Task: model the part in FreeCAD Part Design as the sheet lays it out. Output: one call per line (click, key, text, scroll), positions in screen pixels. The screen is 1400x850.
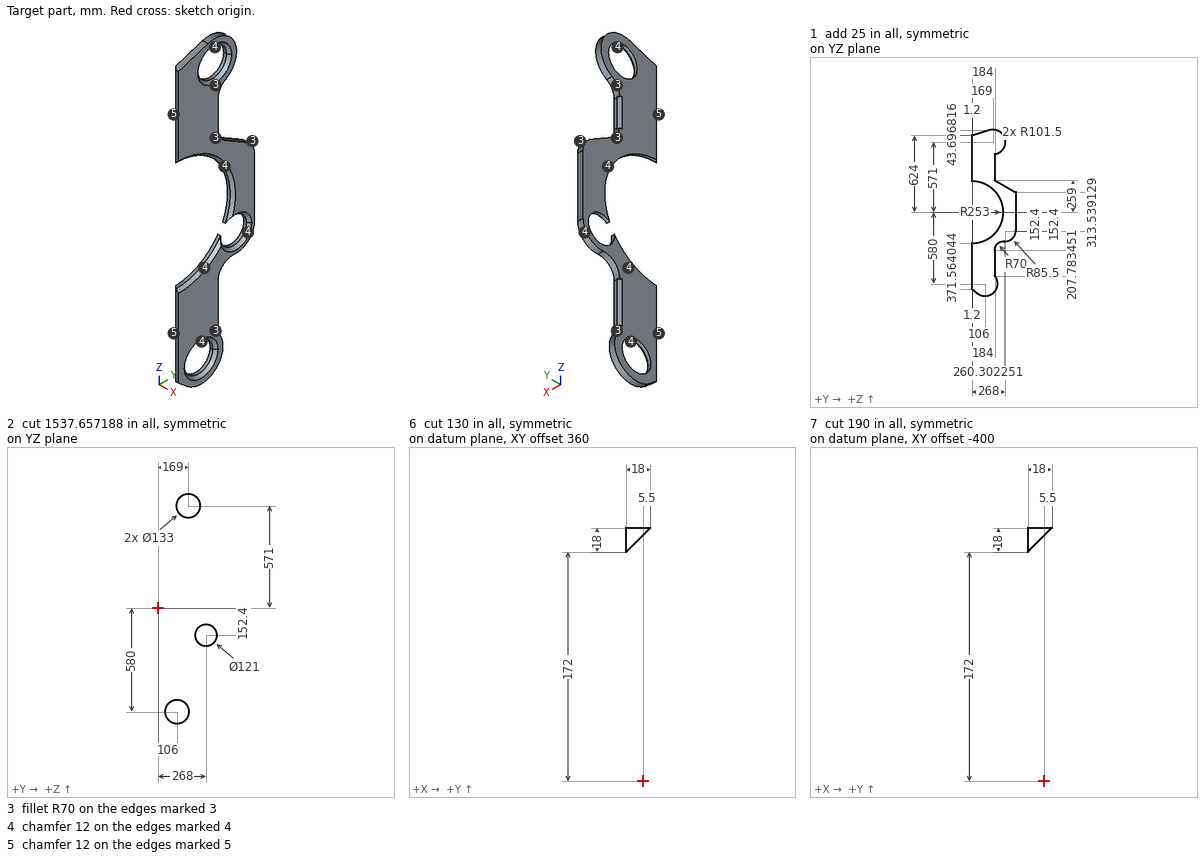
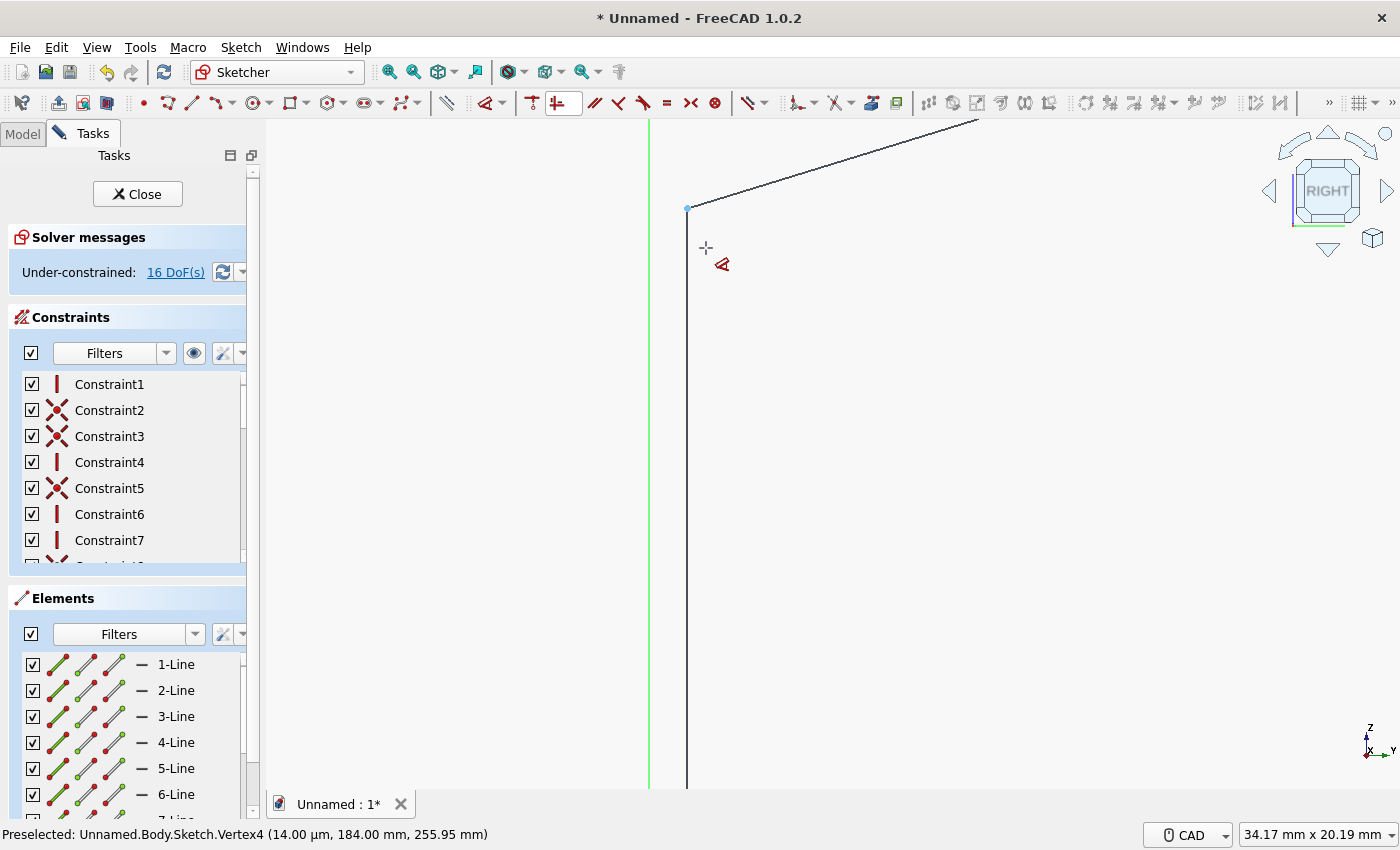
click(687, 209)
click(668, 175)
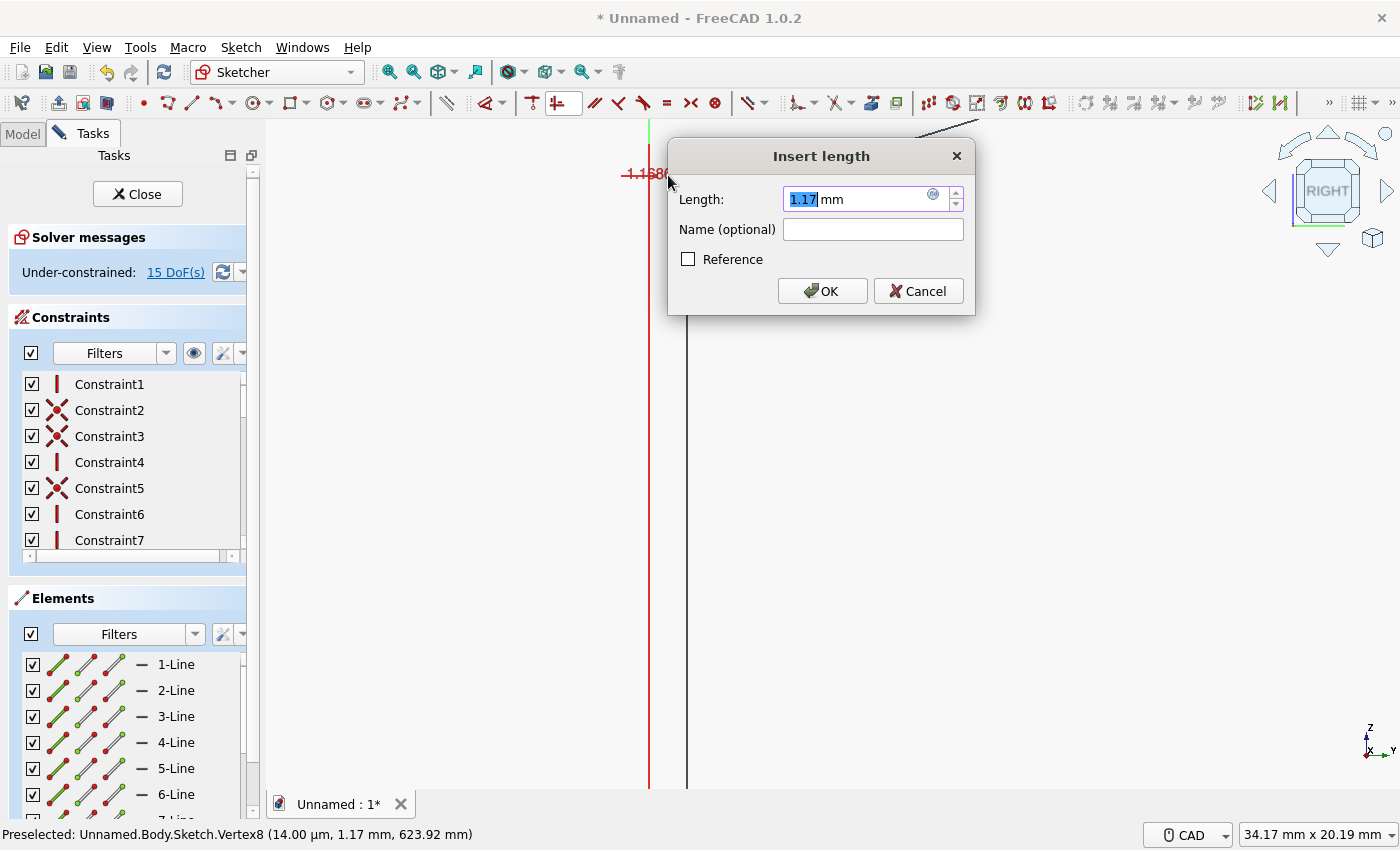
text(1.2)
key(Return)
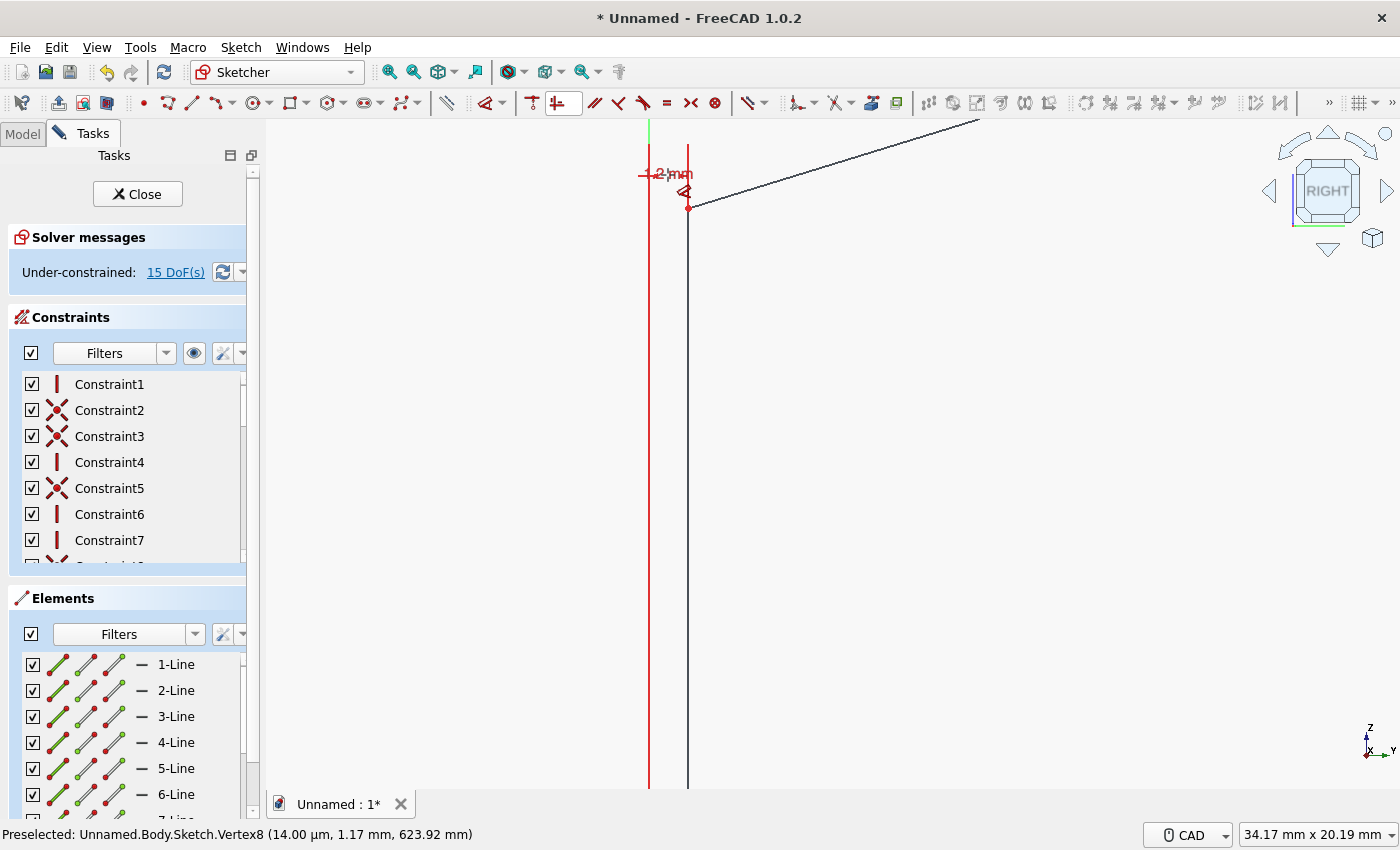
scroll(764, 454, down, 15)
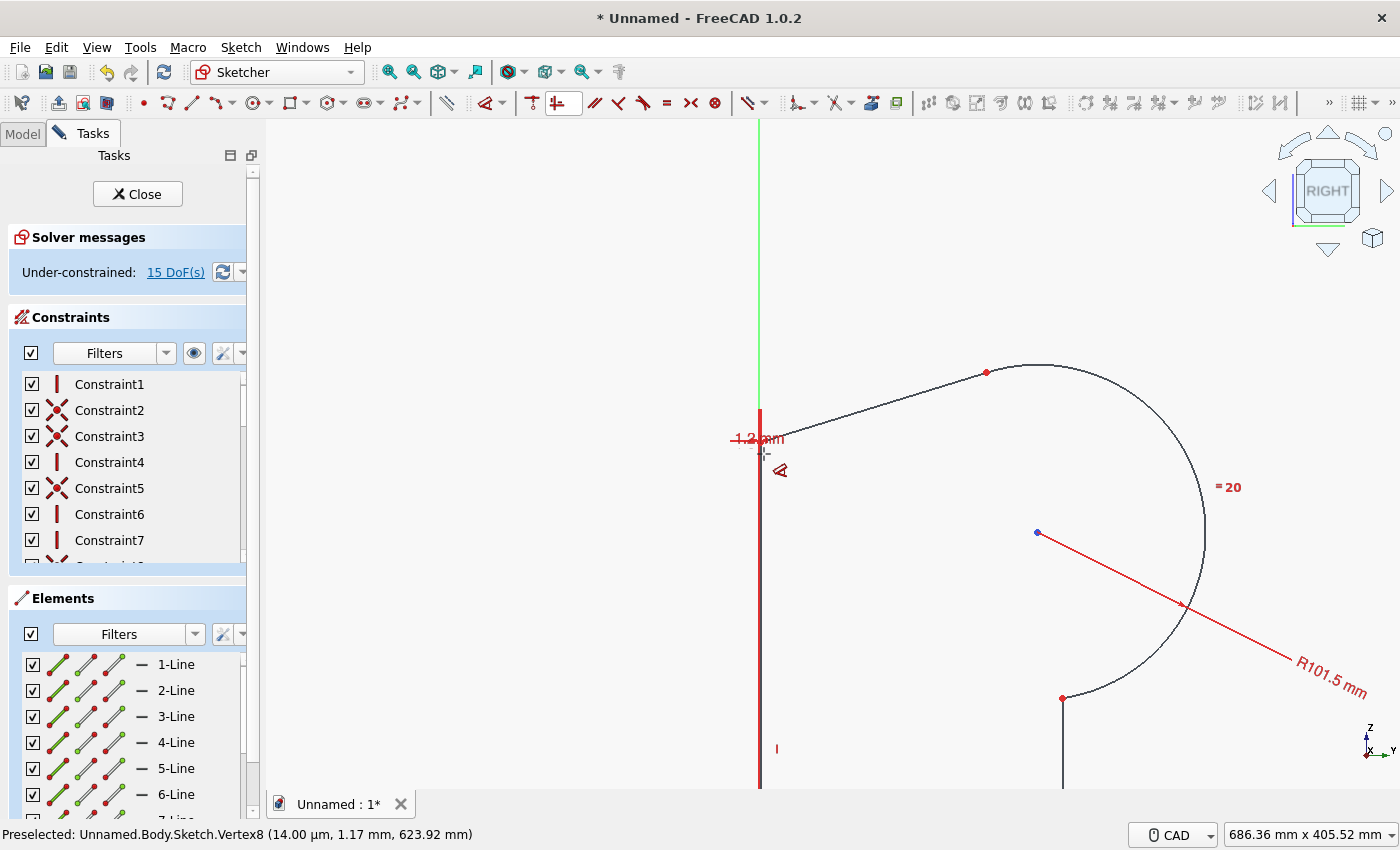
scroll(692, 198, down, 8)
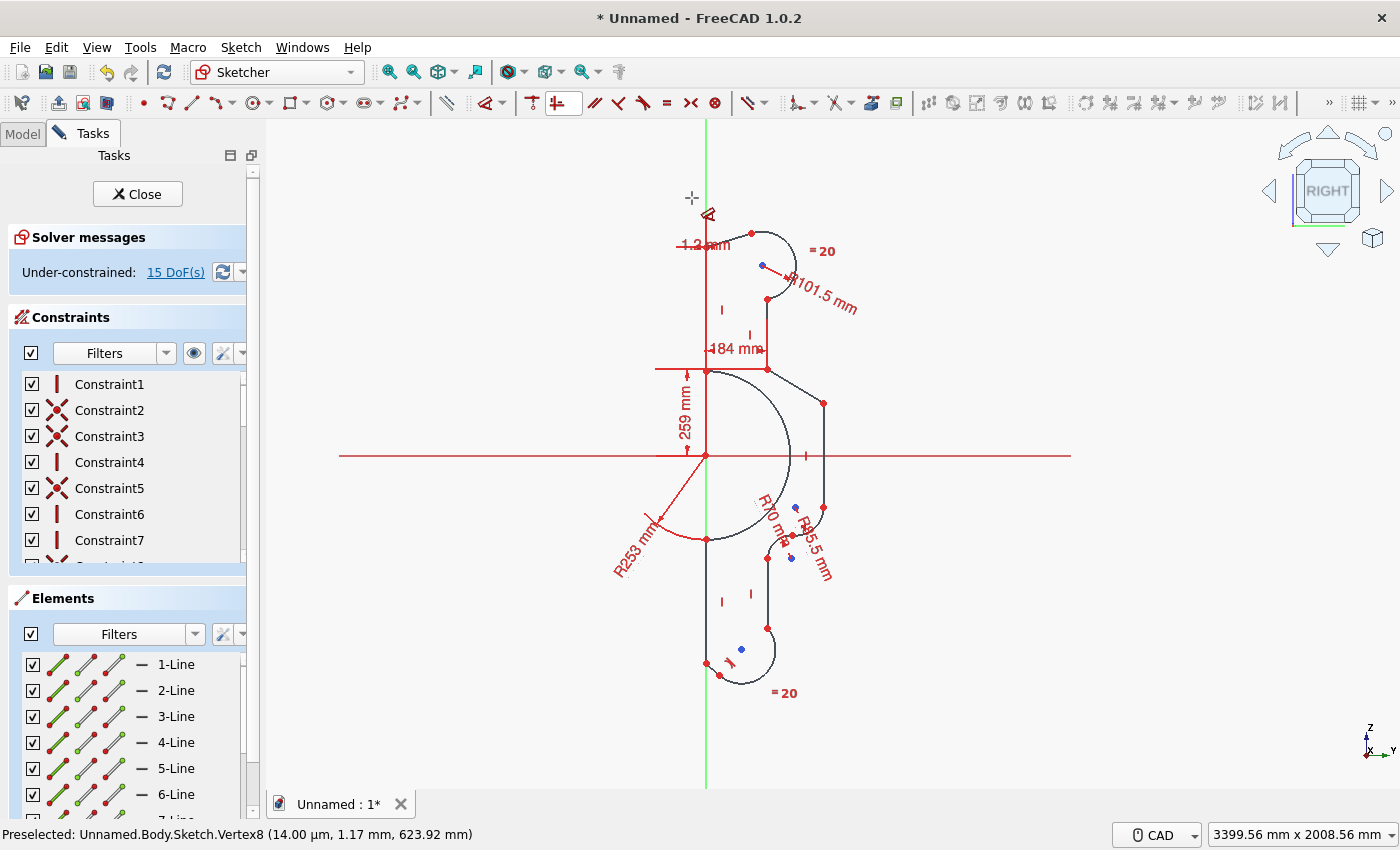
click(706, 247)
click(672, 304)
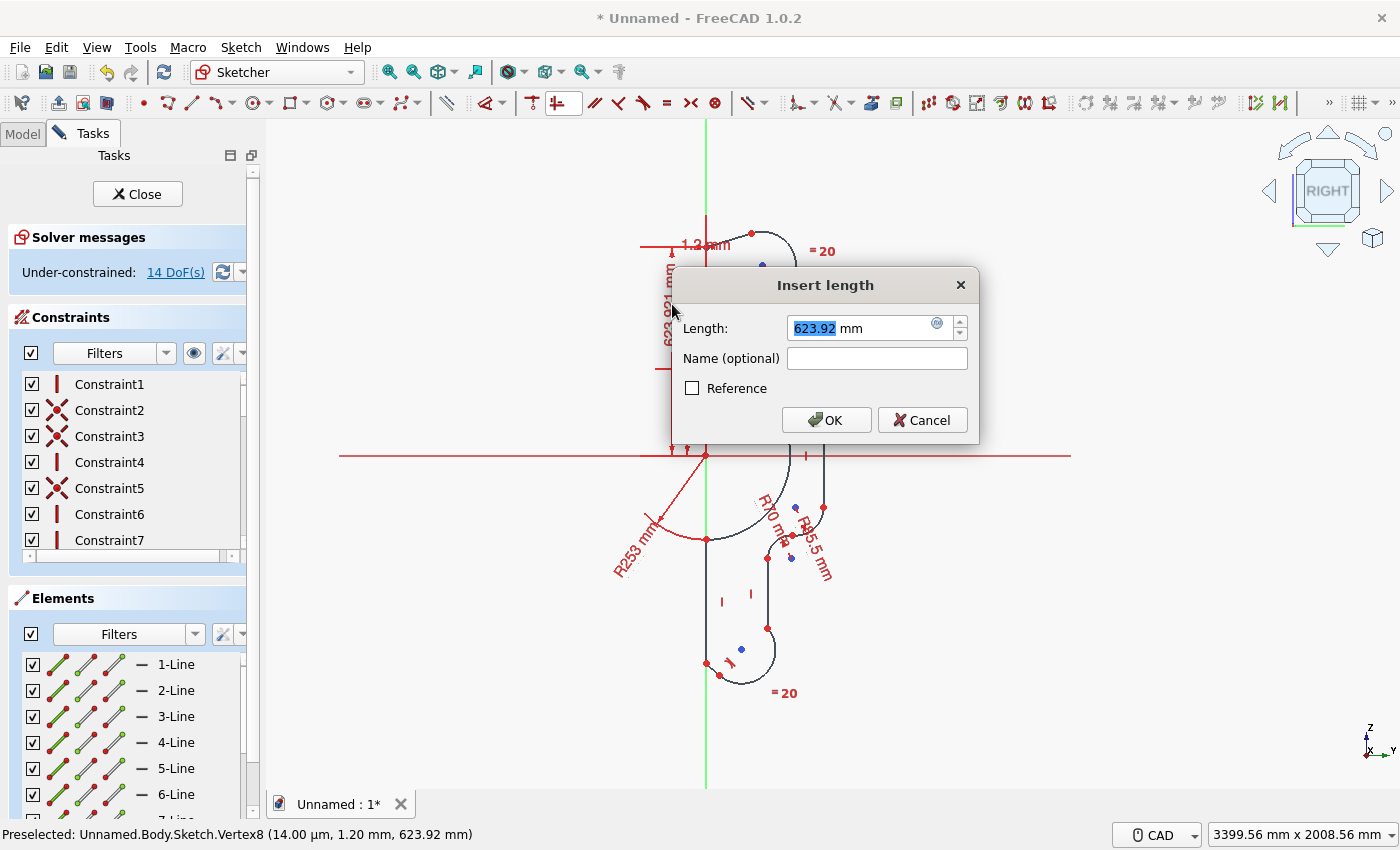
text(624)
key(Return)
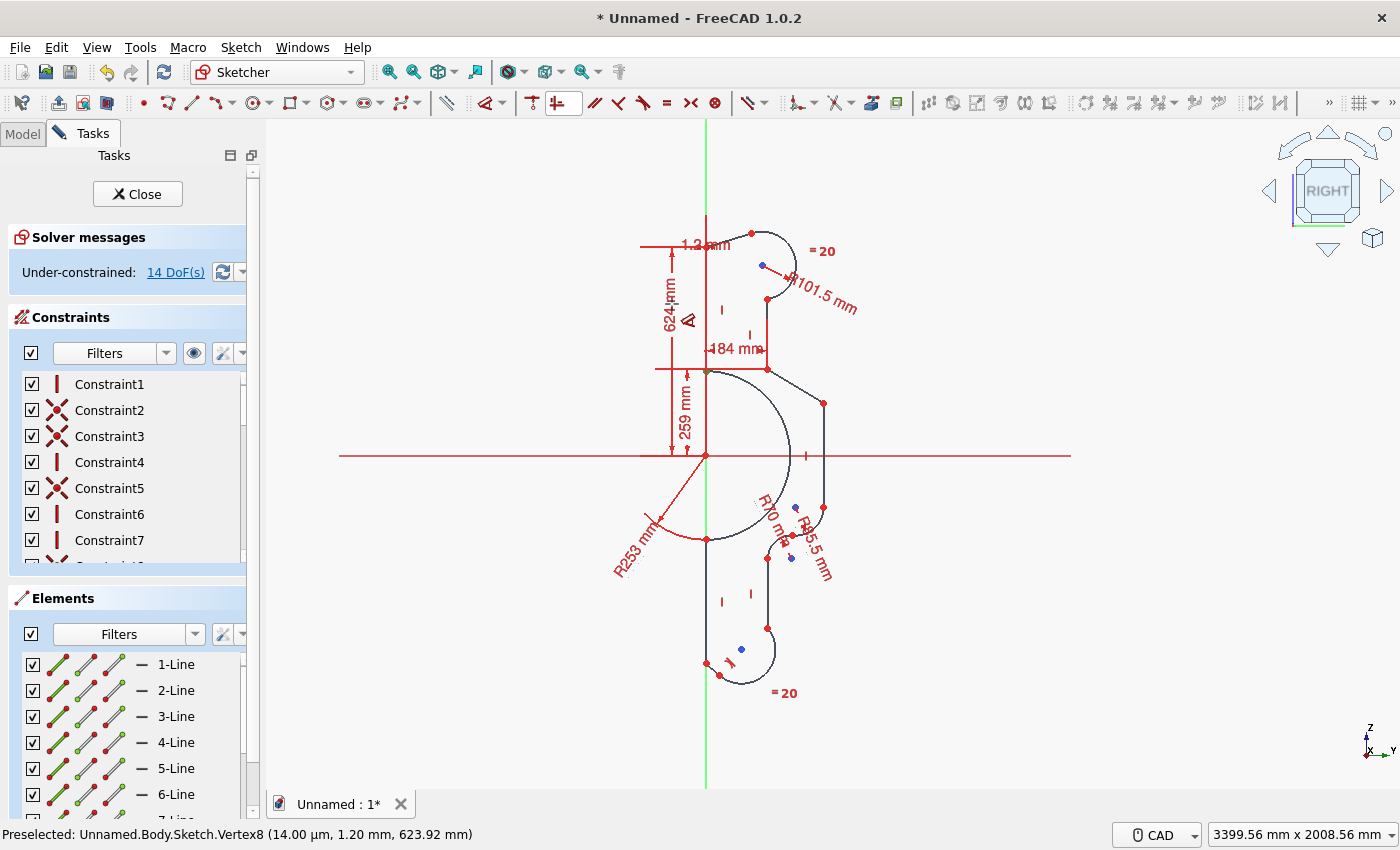
scroll(706, 540, up, 23)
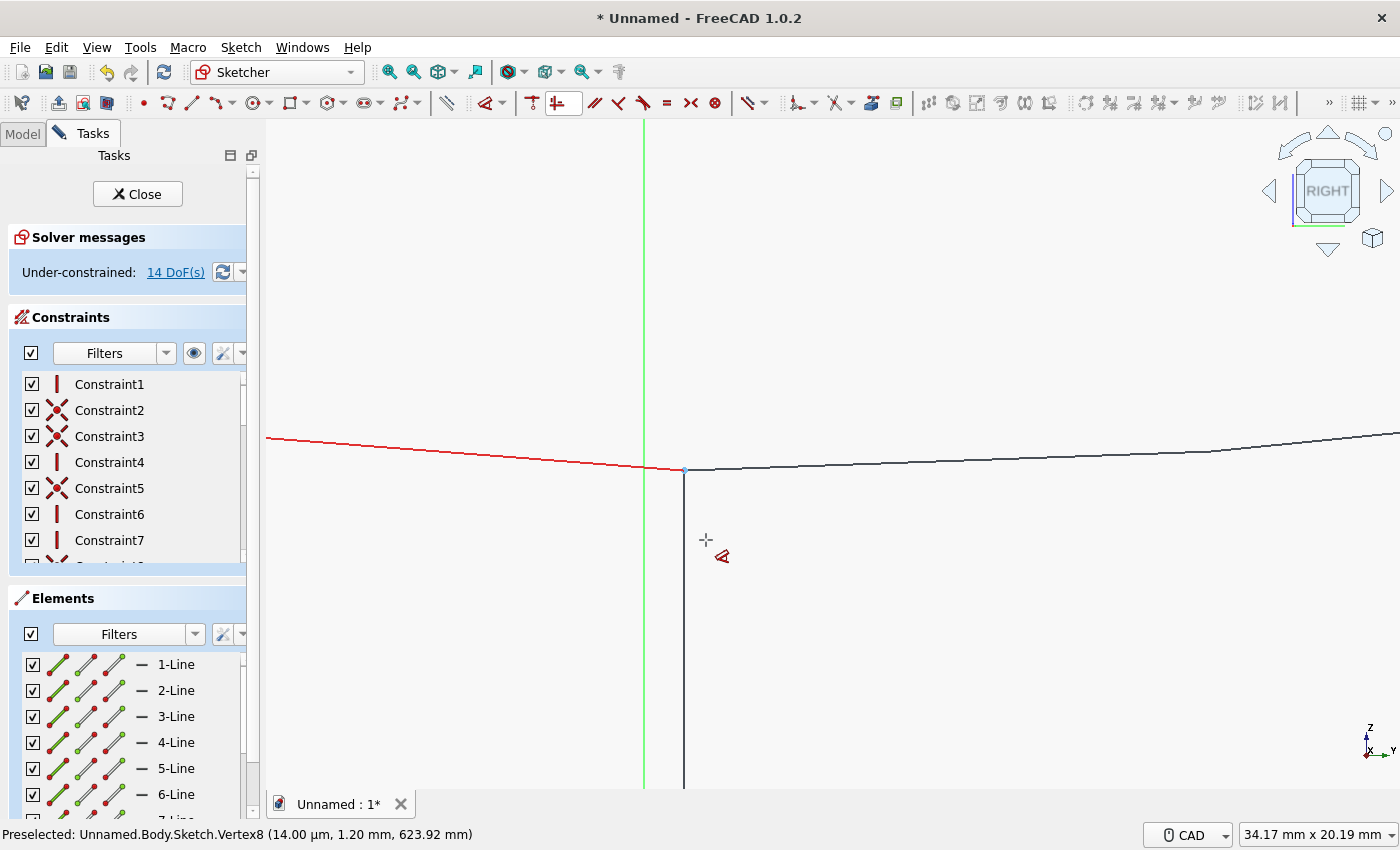
click(684, 471)
click(664, 505)